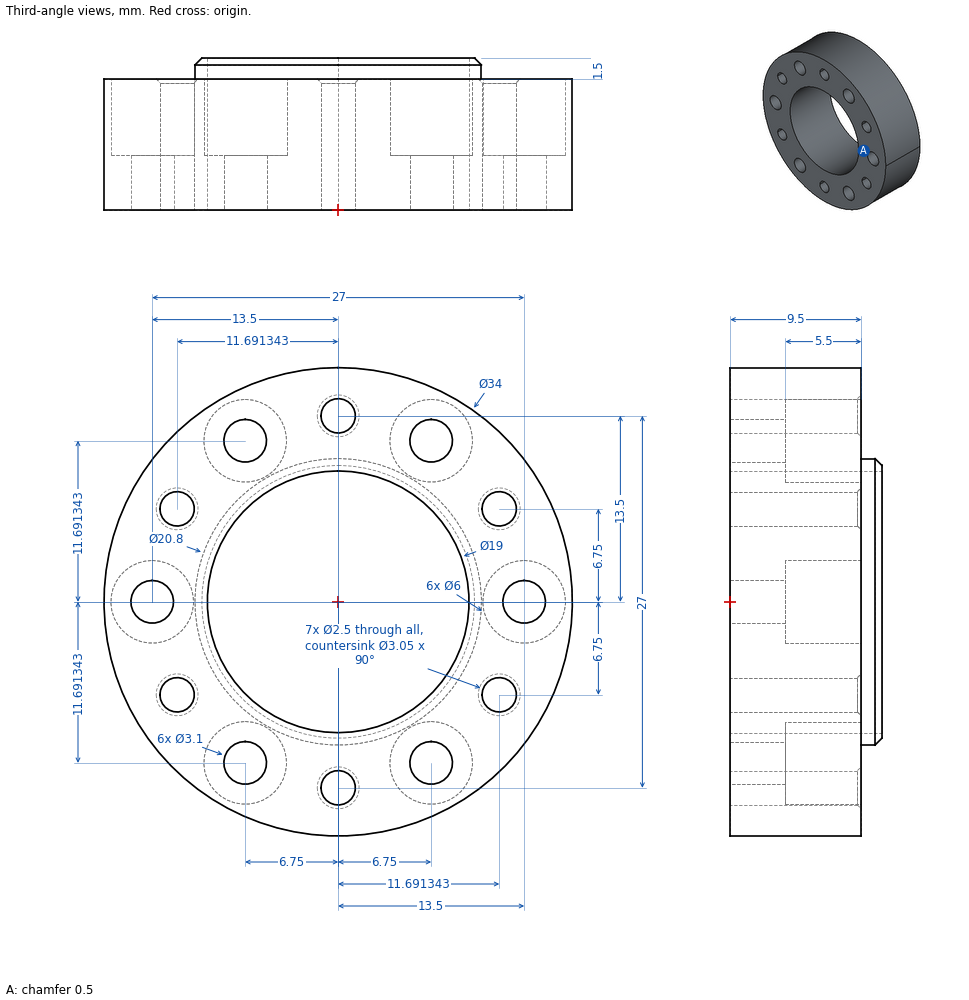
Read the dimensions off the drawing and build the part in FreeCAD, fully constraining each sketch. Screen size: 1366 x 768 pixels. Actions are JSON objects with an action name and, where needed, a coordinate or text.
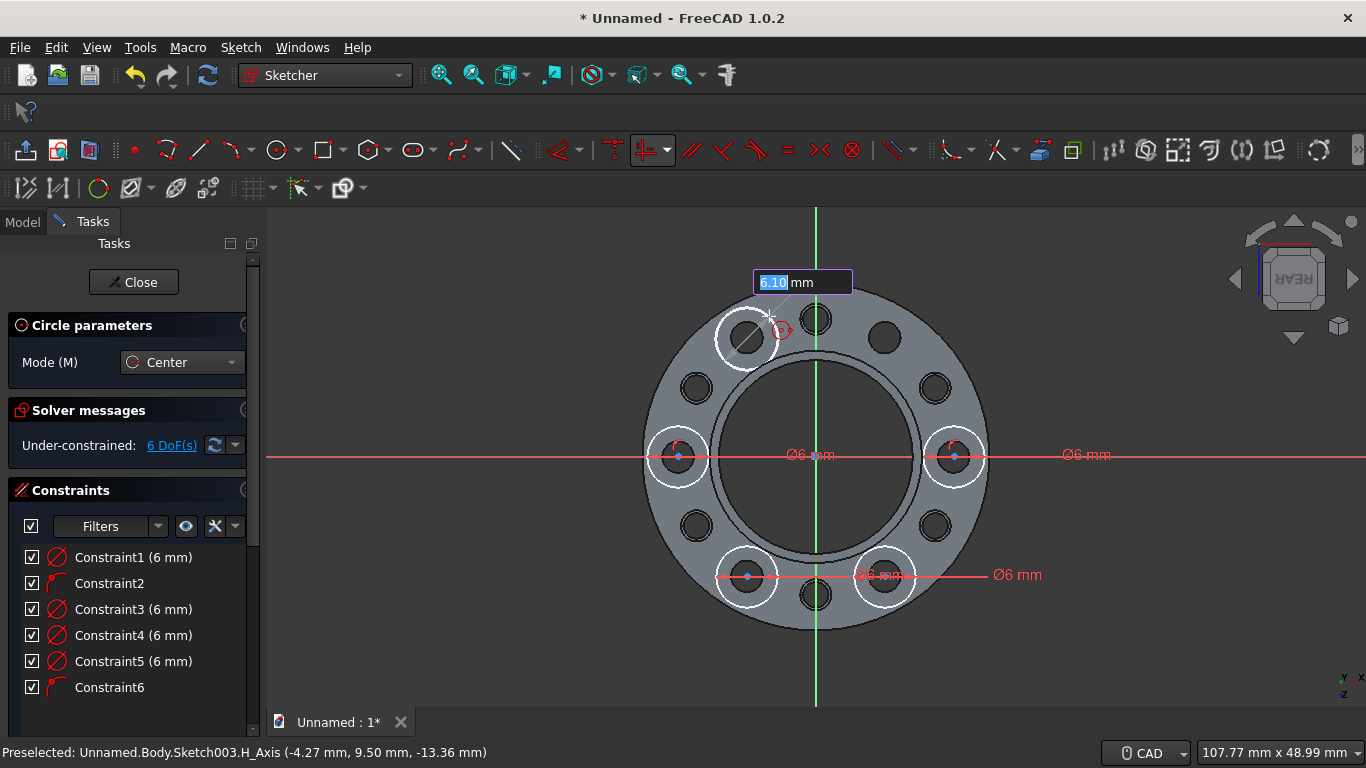
{"action": "type", "text": "6"}
{"action": "key", "text": "Return"}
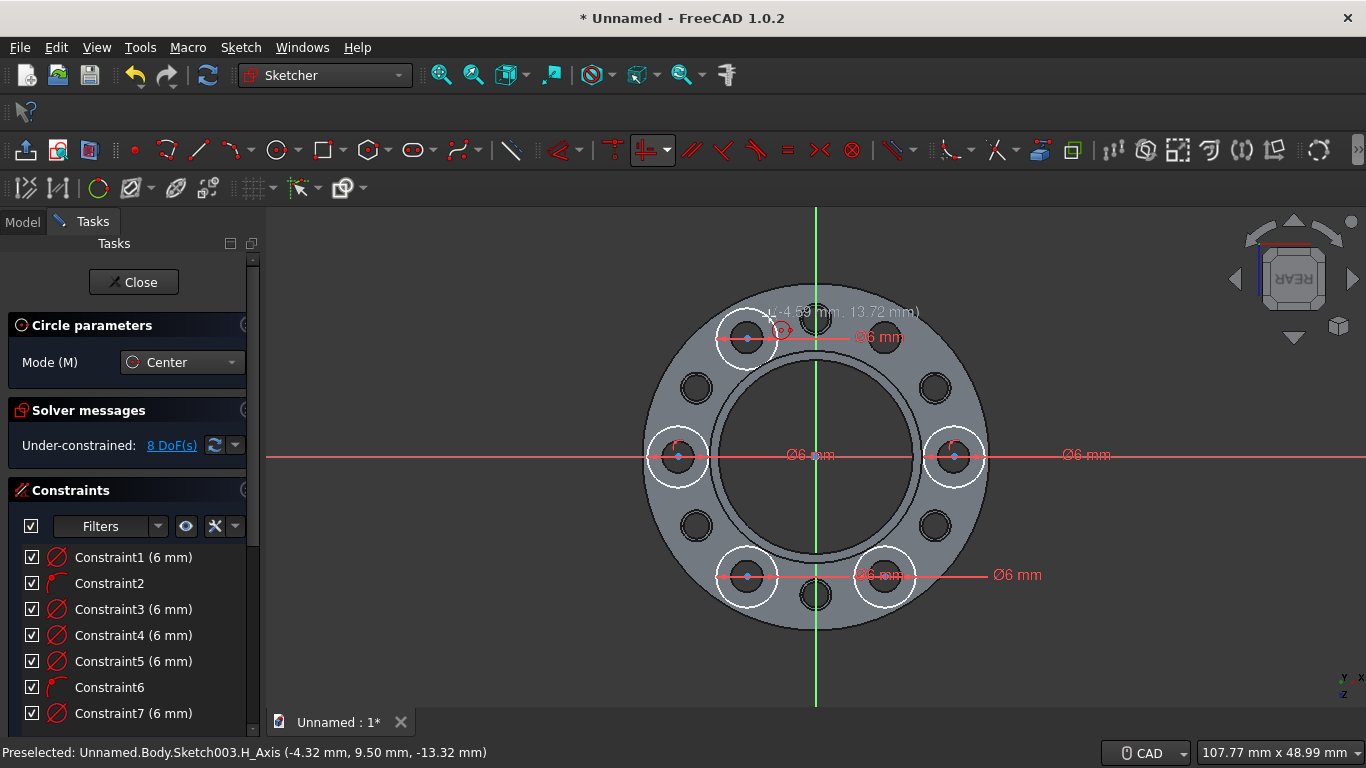
{"action": "left_click", "coordinate": [885, 338]}
{"action": "mouse_move", "coordinate": [906, 316]}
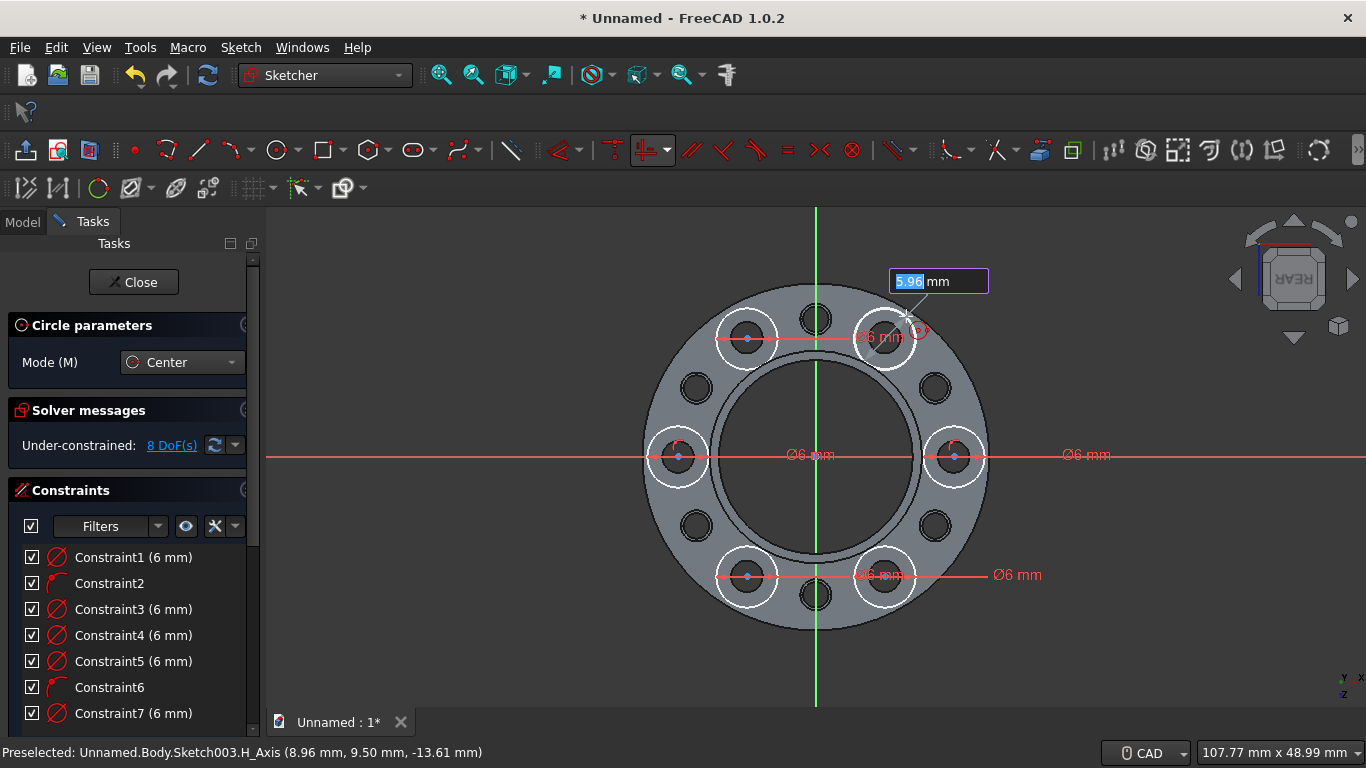
{"action": "type", "text": "6"}
{"action": "key", "text": "Return"}
{"action": "key", "text": "Escape"}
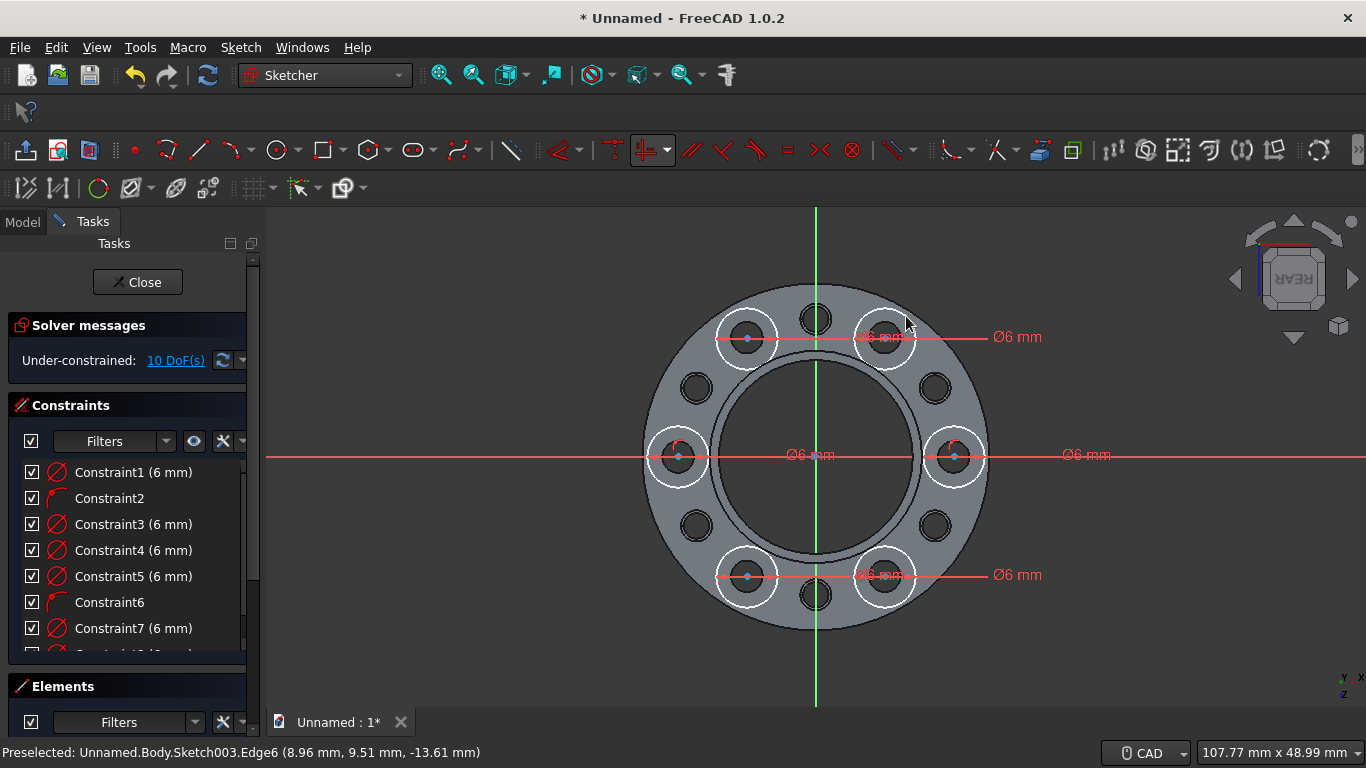
{"action": "left_click", "coordinate": [885, 577]}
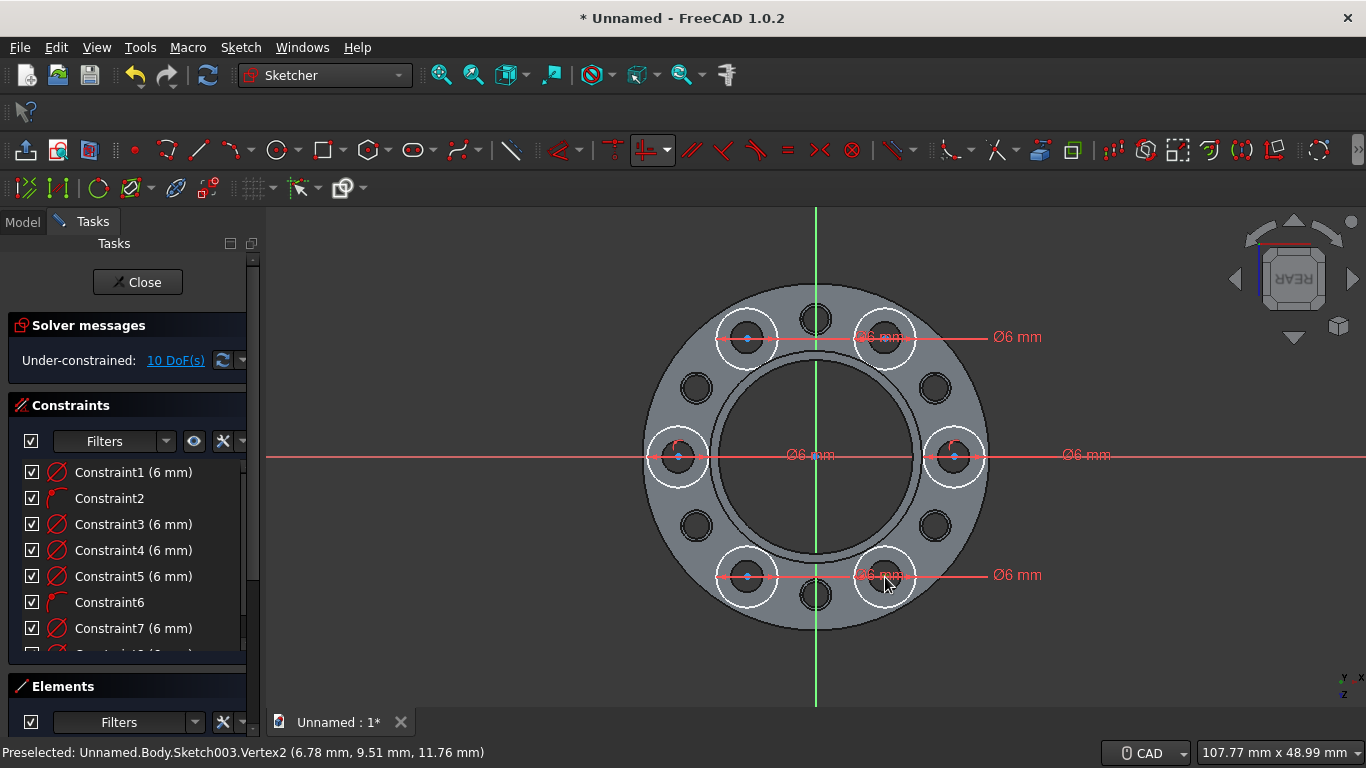
{"action": "left_click", "coordinate": [747, 577]}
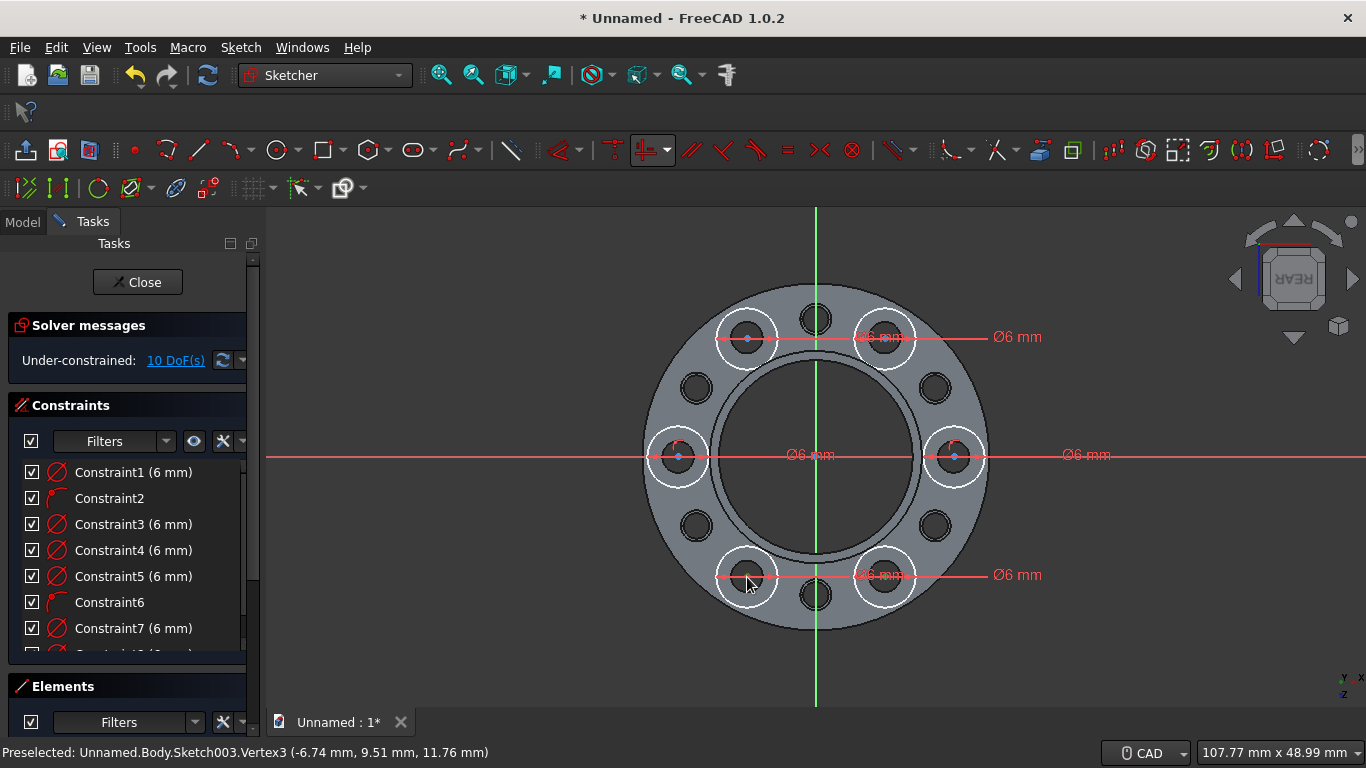
{"action": "left_click", "coordinate": [670, 150]}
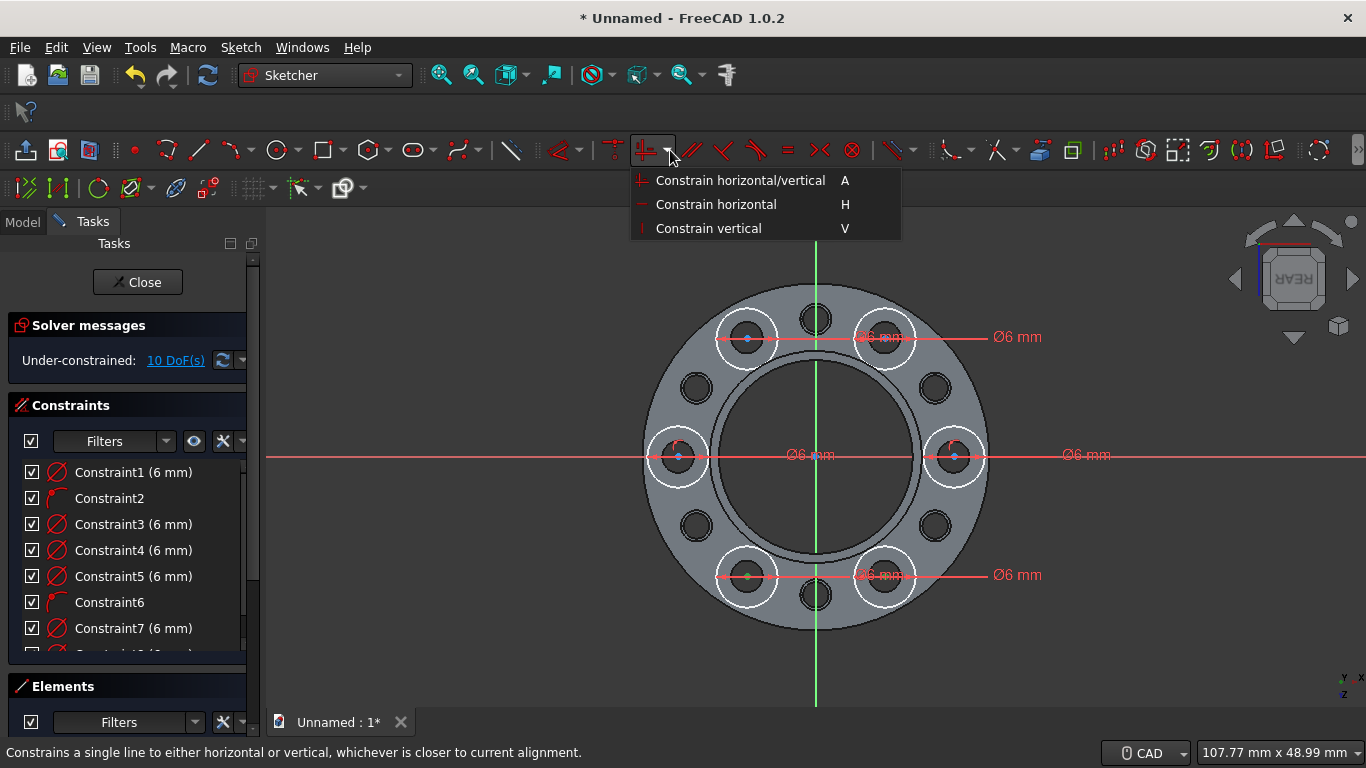
{"action": "left_click", "coordinate": [766, 204]}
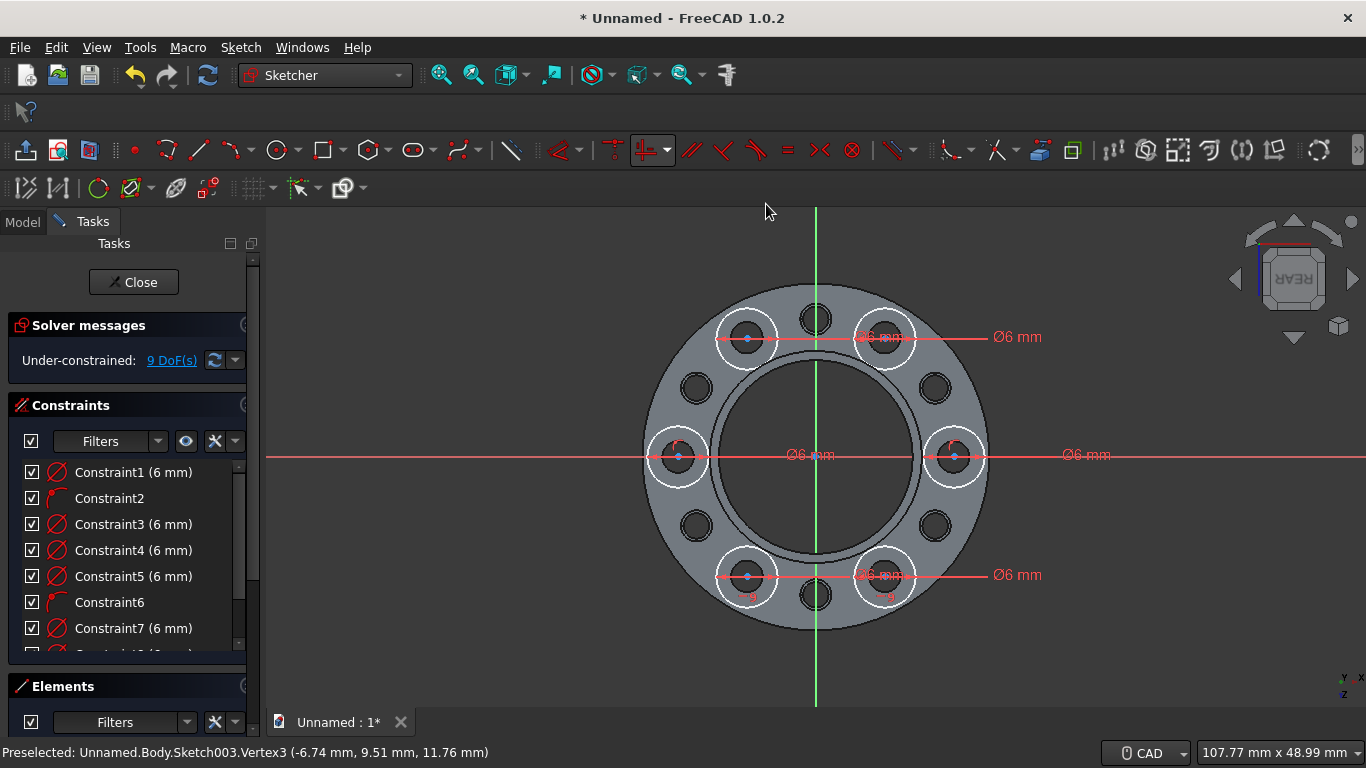
{"action": "left_click", "coordinate": [747, 577]}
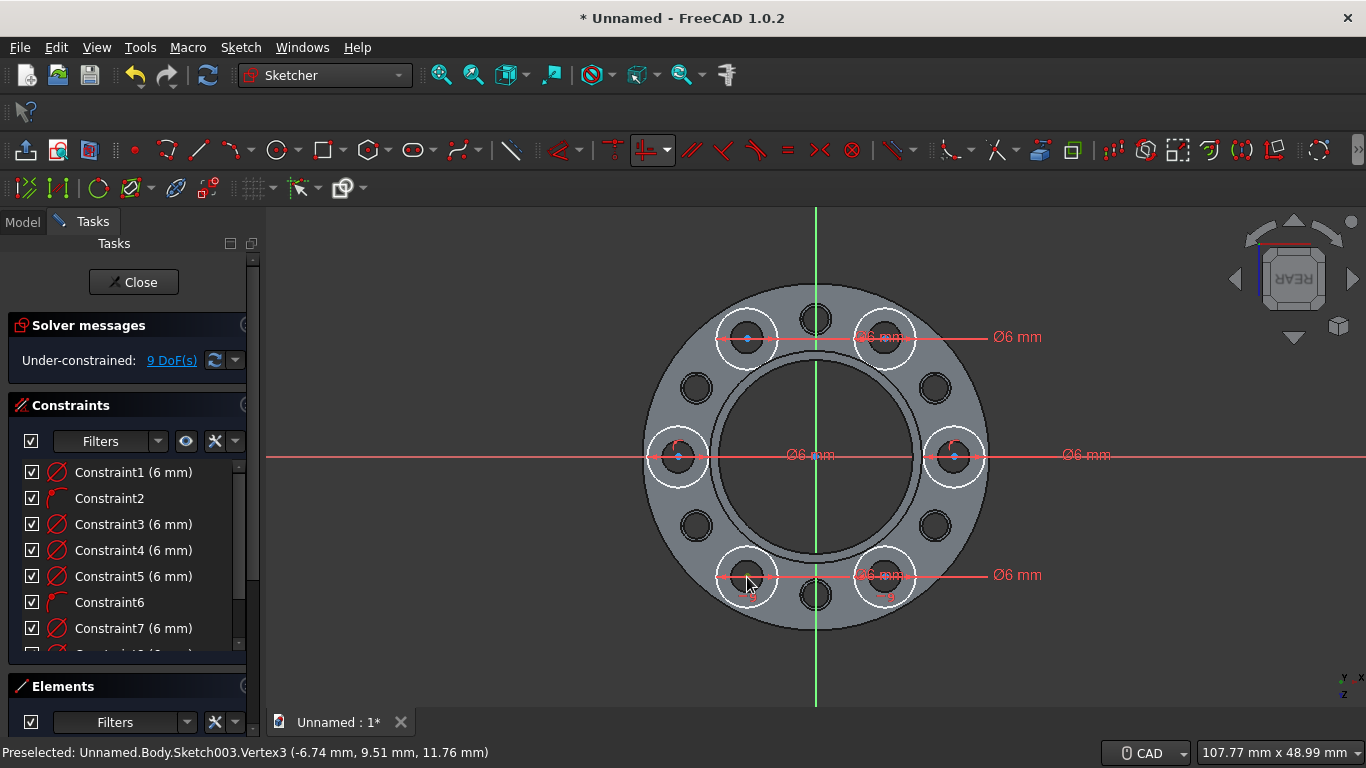
{"action": "left_click", "coordinate": [747, 339]}